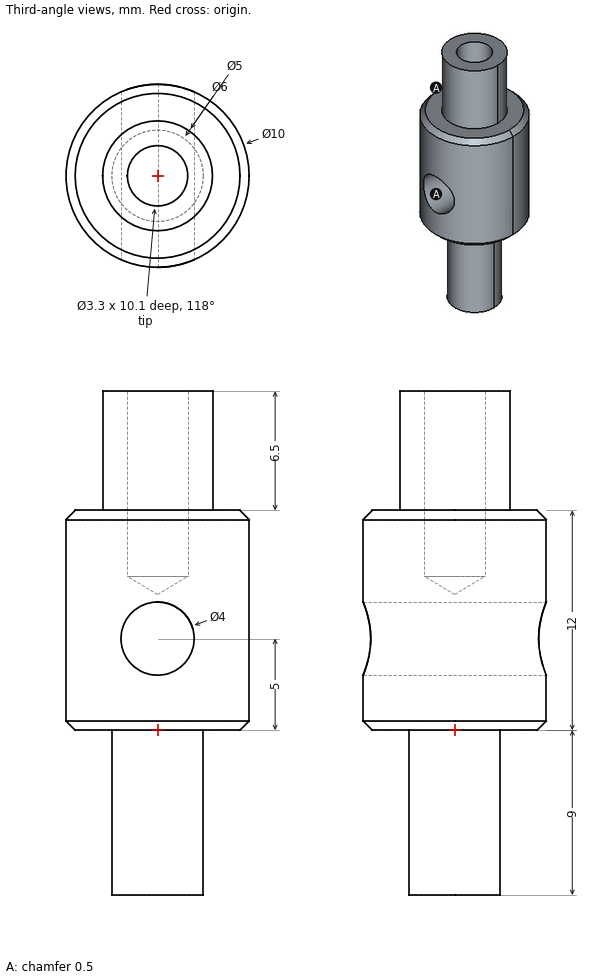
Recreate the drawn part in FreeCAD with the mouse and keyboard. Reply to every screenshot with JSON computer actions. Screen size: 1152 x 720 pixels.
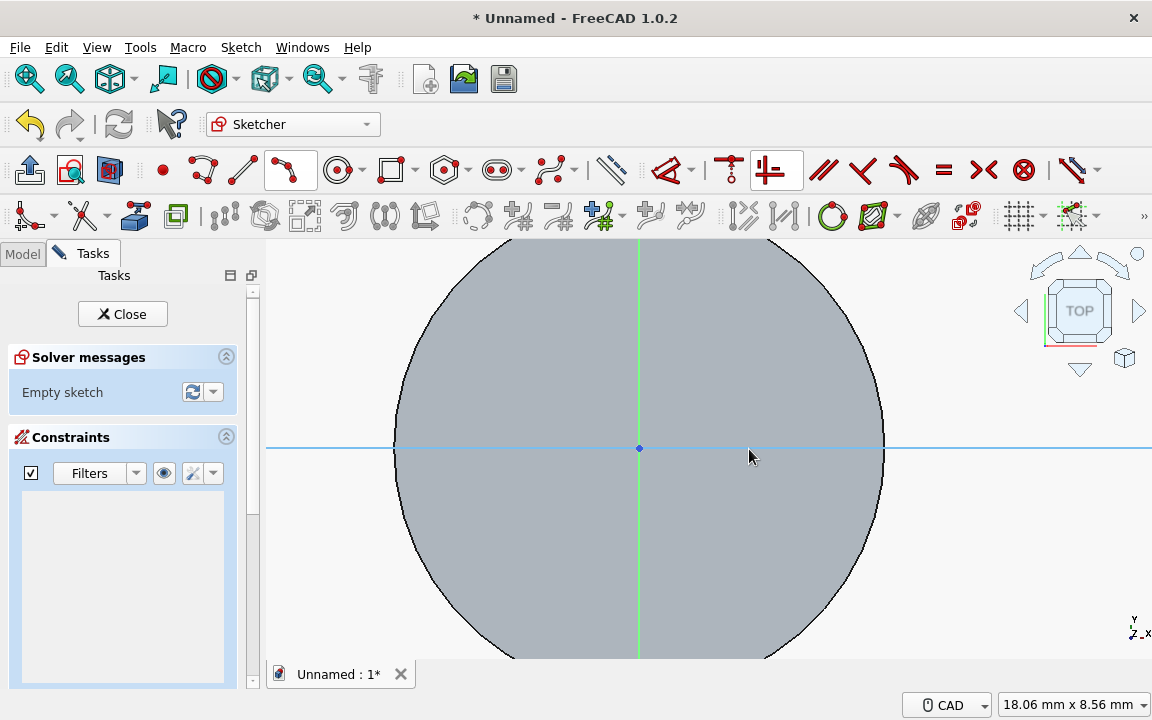
{"action": "left_click", "coordinate": [338, 170]}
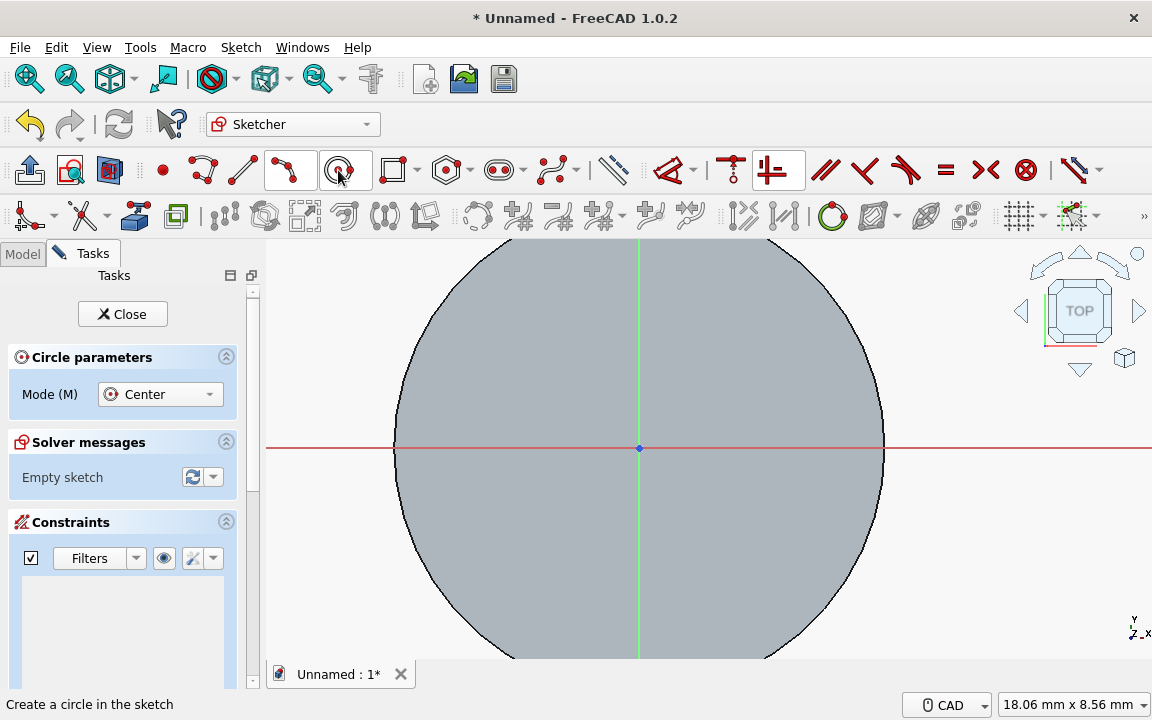
{"action": "left_click", "coordinate": [639, 448]}
{"action": "left_click", "coordinate": [726, 361]}
{"action": "key", "text": "Escape"}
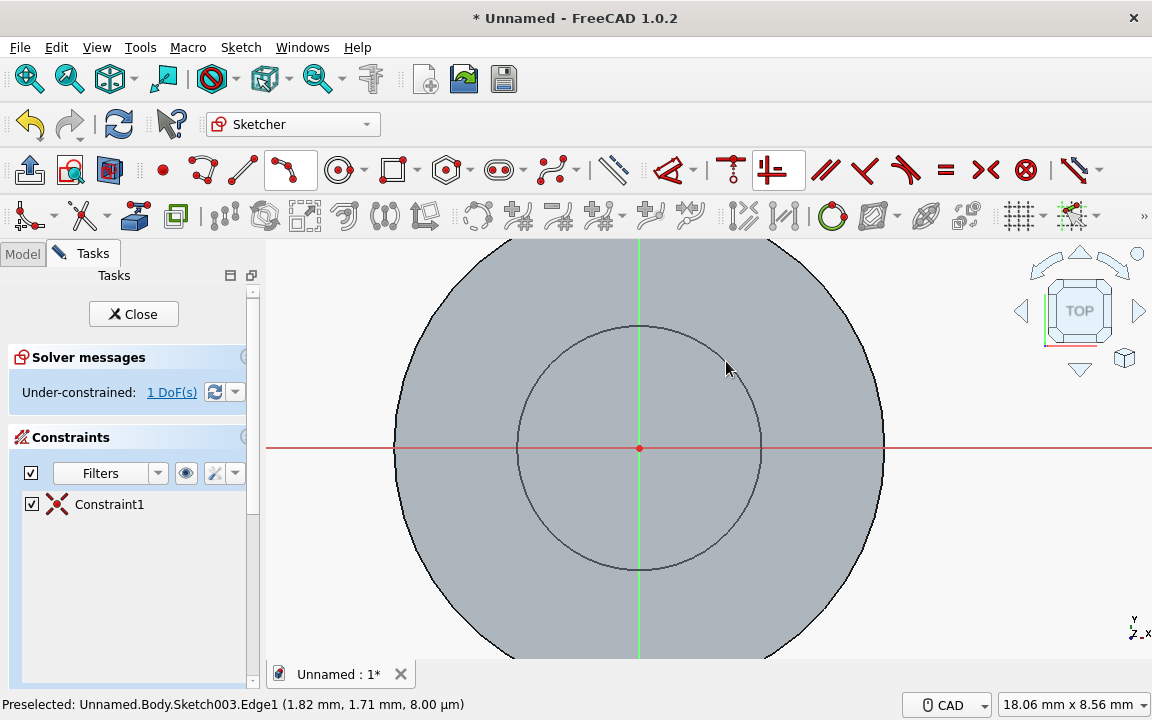
{"action": "key", "text": "d"}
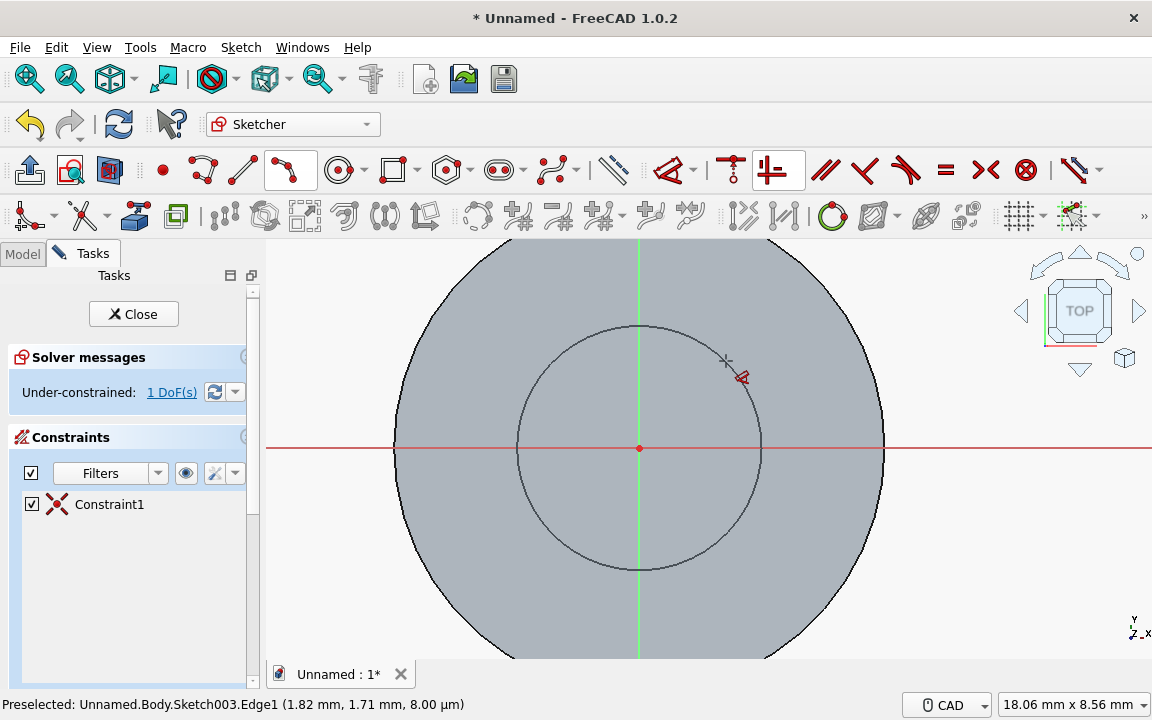
{"action": "left_click", "coordinate": [725, 361]}
{"action": "left_click", "coordinate": [747, 338]}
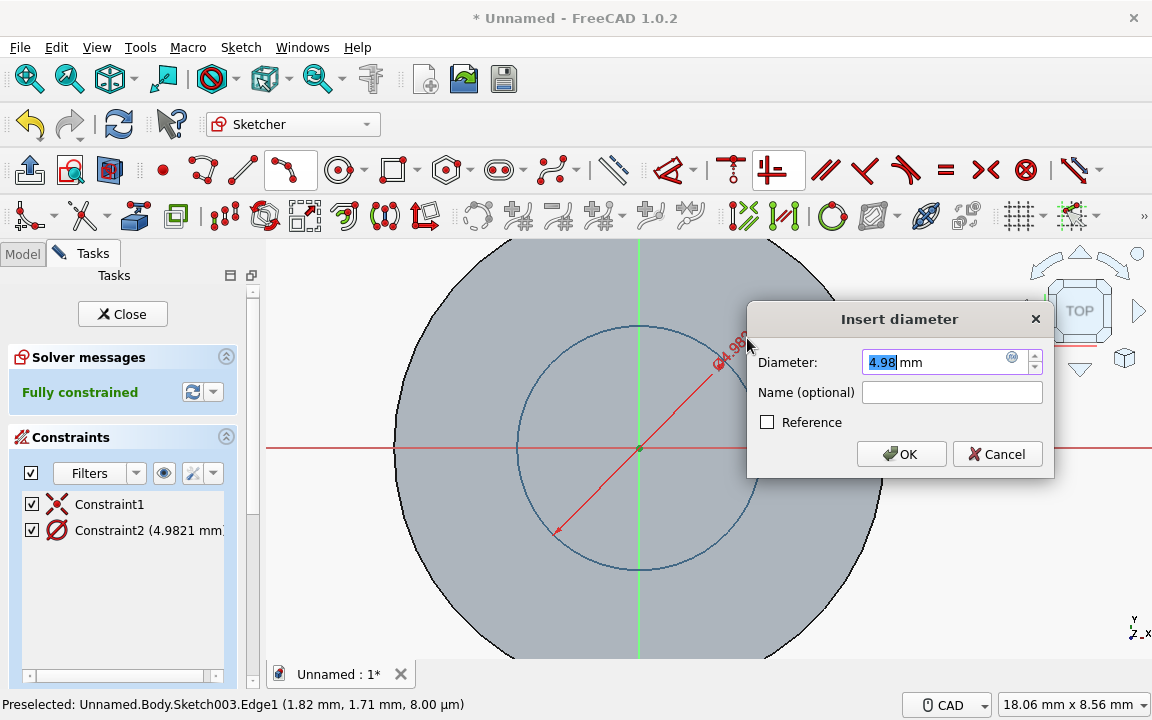
{"action": "type", "text": "5"}
{"action": "key", "text": "Return"}
{"action": "key", "text": "Escape"}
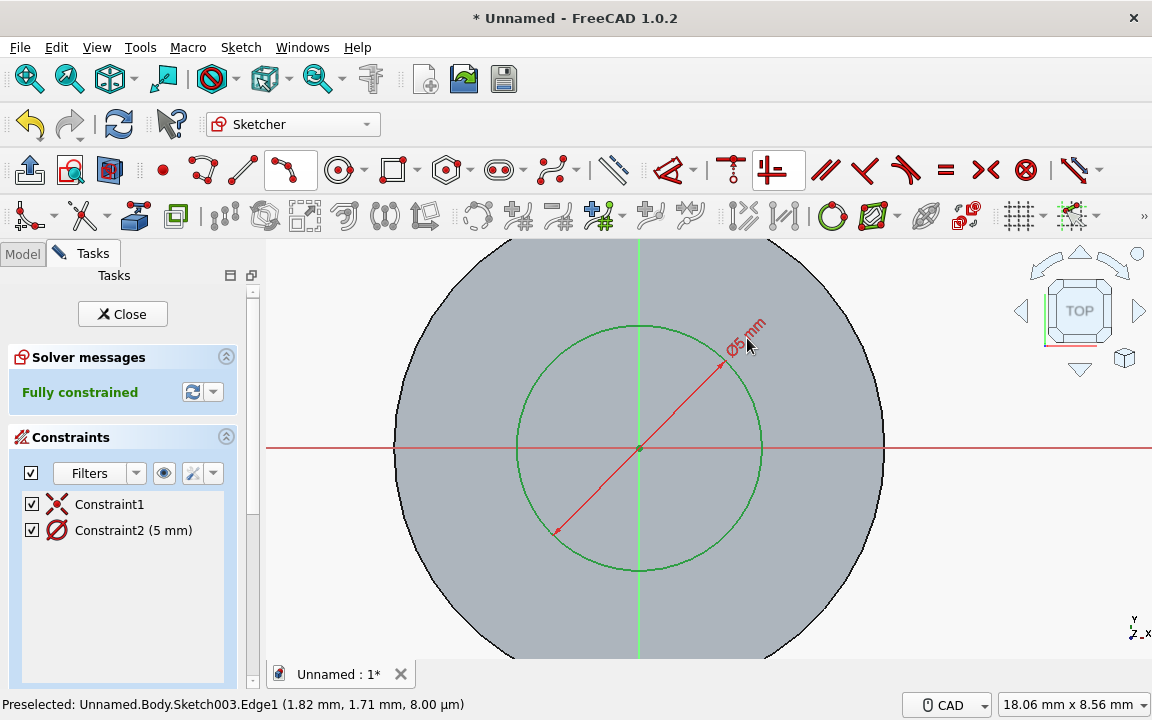
{"action": "left_click", "coordinate": [123, 314]}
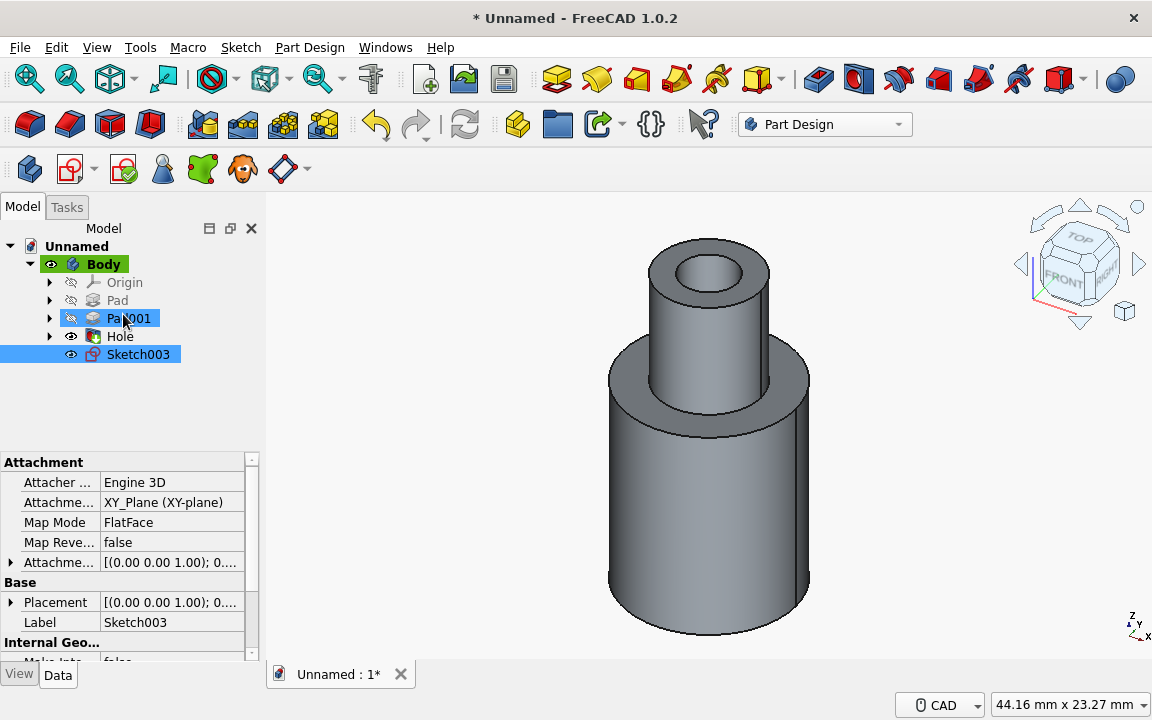
{"action": "left_click", "coordinate": [558, 80]}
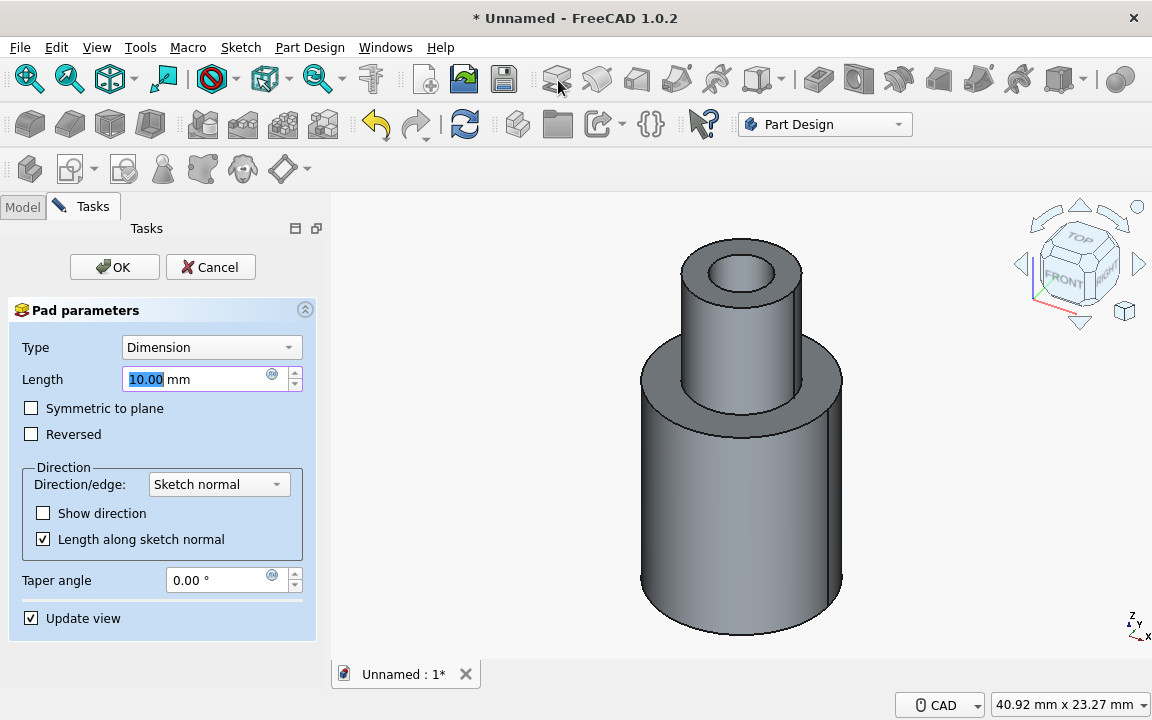
{"action": "type", "text": "9"}
{"action": "key", "text": "Tab"}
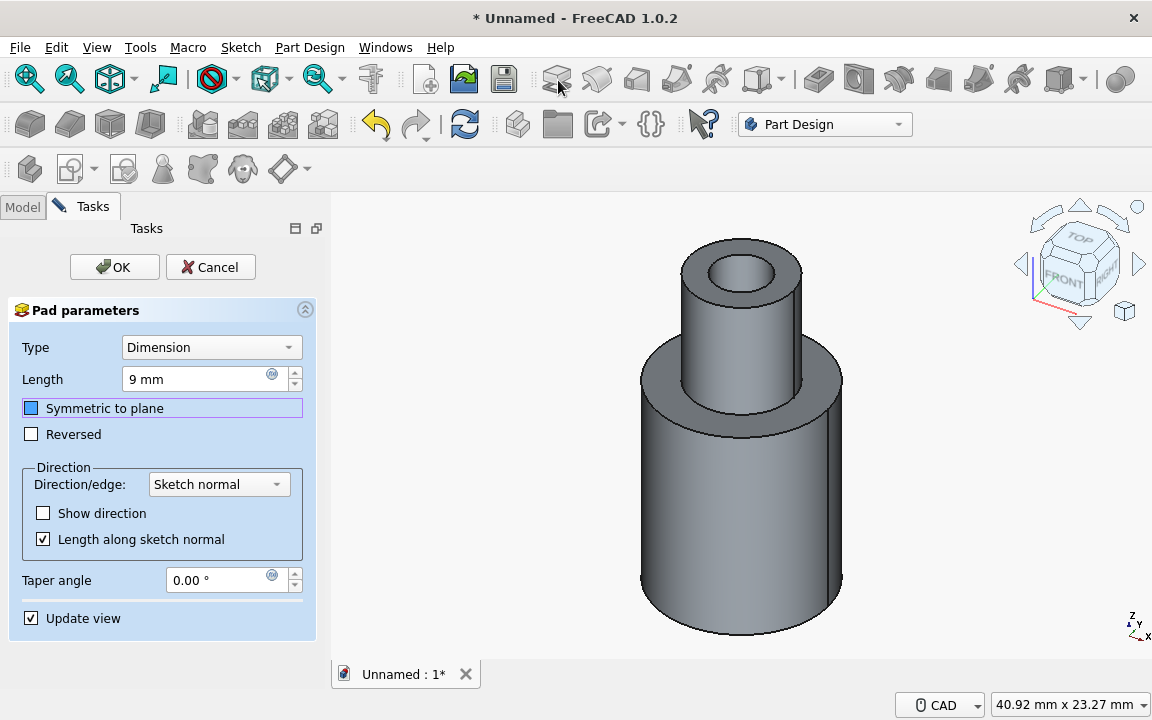
{"action": "left_click", "coordinate": [30, 434]}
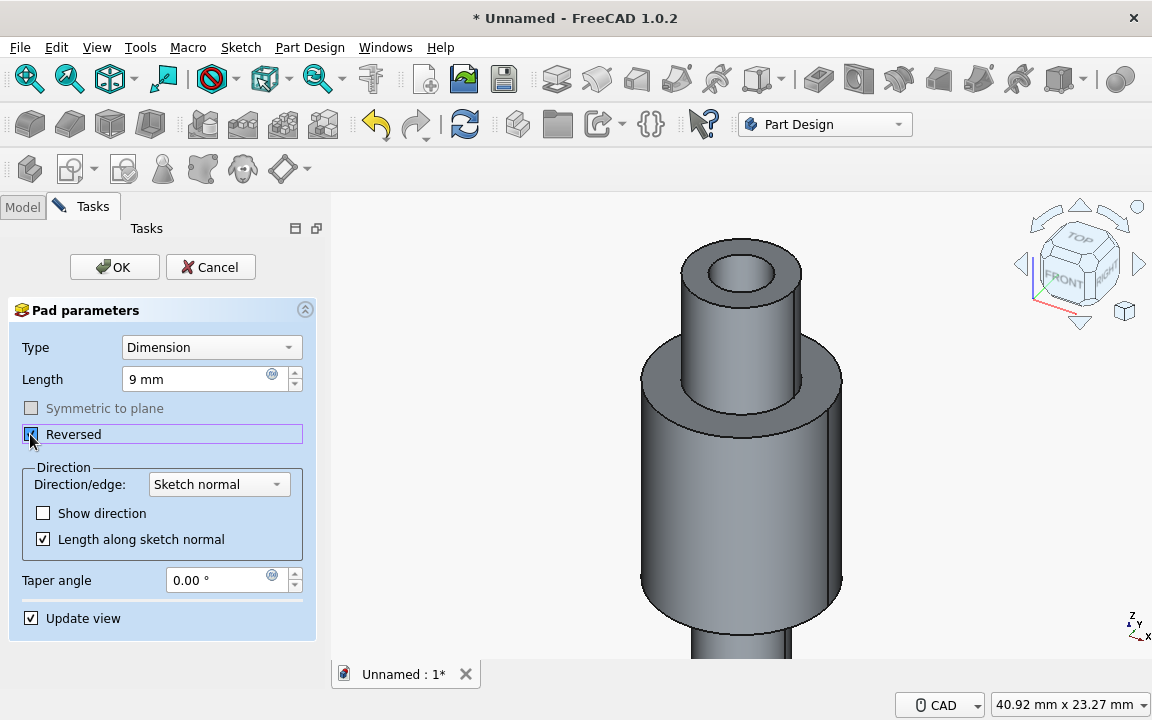
{"action": "left_click", "coordinate": [115, 267]}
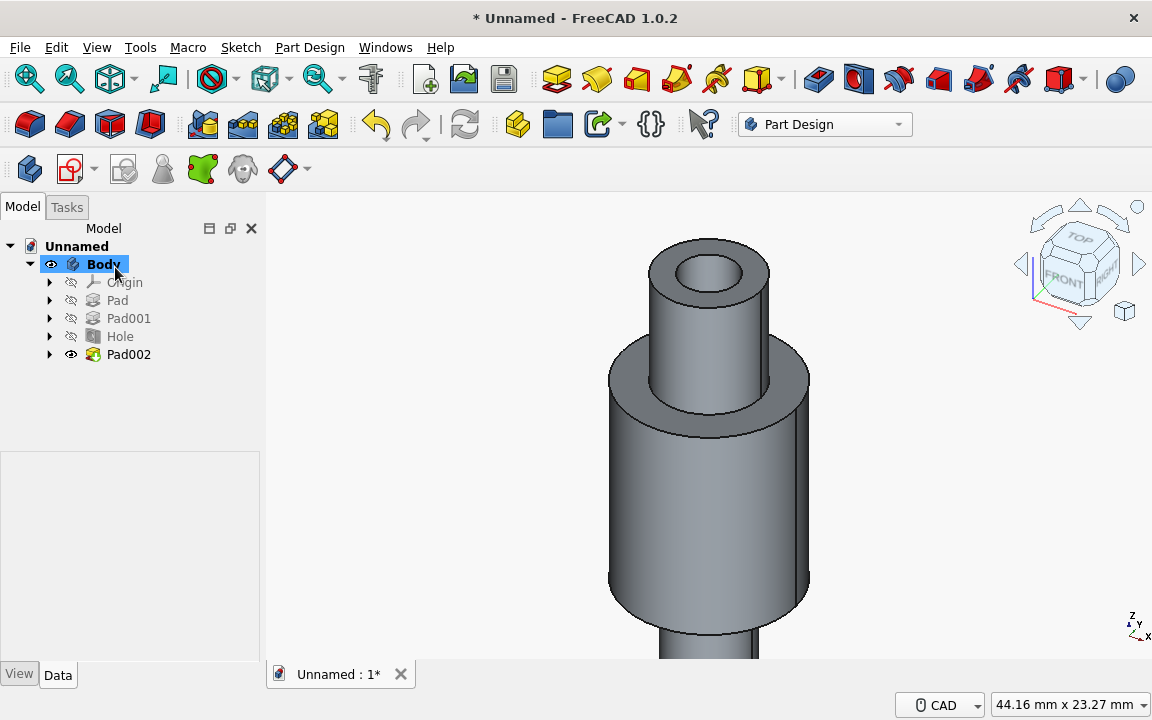
{"action": "left_click", "coordinate": [30, 80]}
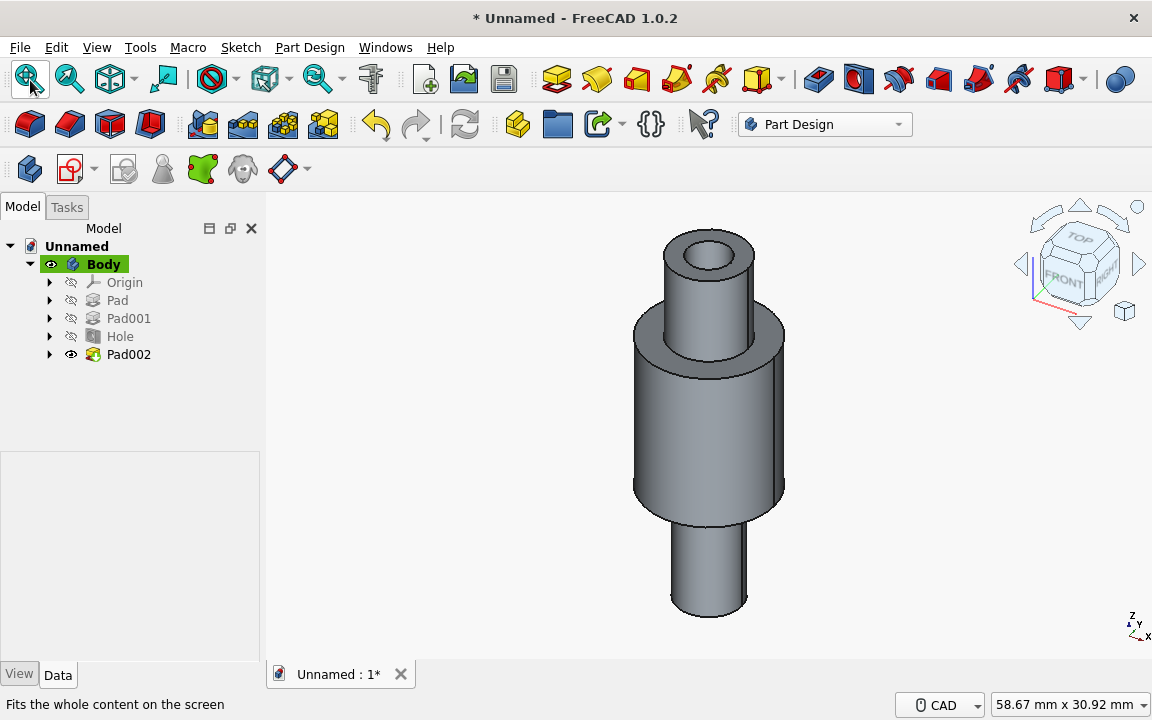
{"action": "left_click", "coordinate": [70, 170]}